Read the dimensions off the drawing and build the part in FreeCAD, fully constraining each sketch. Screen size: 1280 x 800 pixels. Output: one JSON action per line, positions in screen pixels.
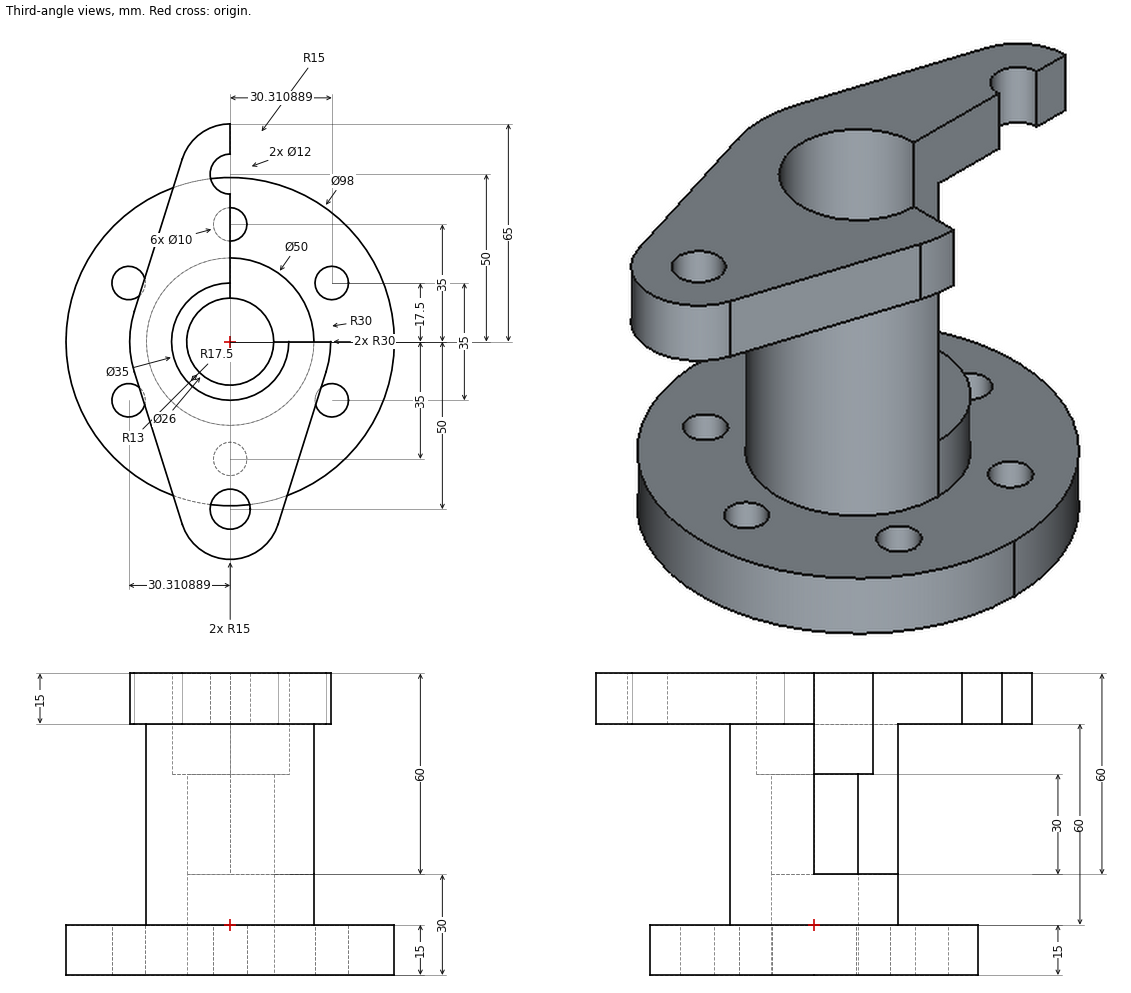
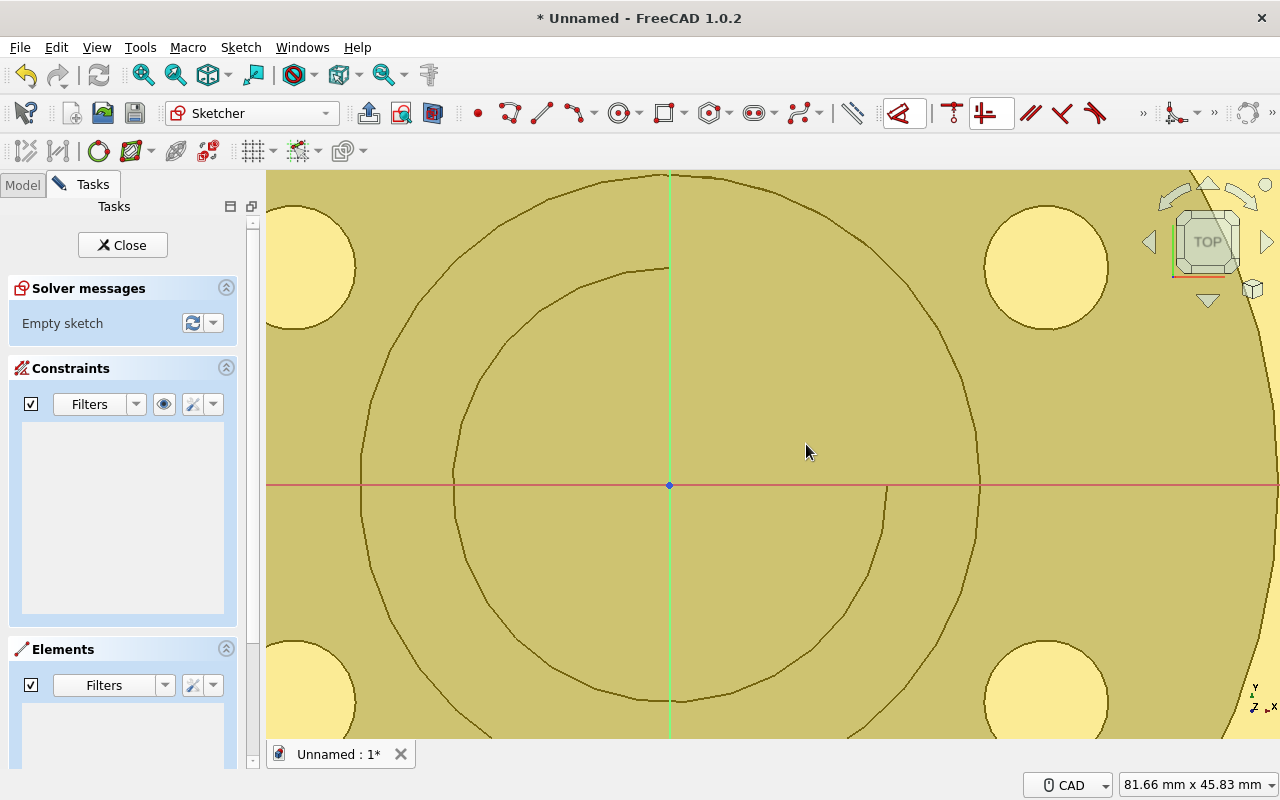
{"action": "left_click", "coordinate": [542, 114]}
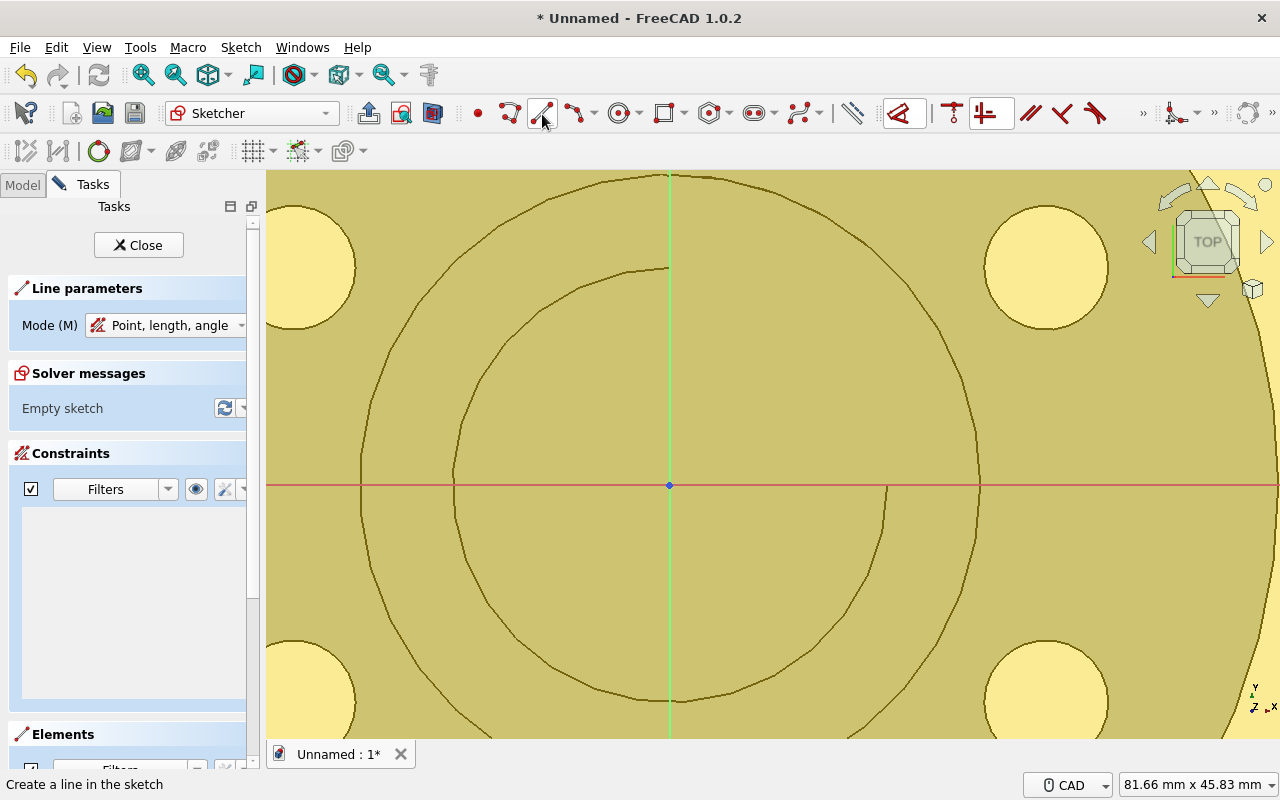
{"action": "left_click", "coordinate": [670, 324]}
{"action": "left_click", "coordinate": [679, 268]}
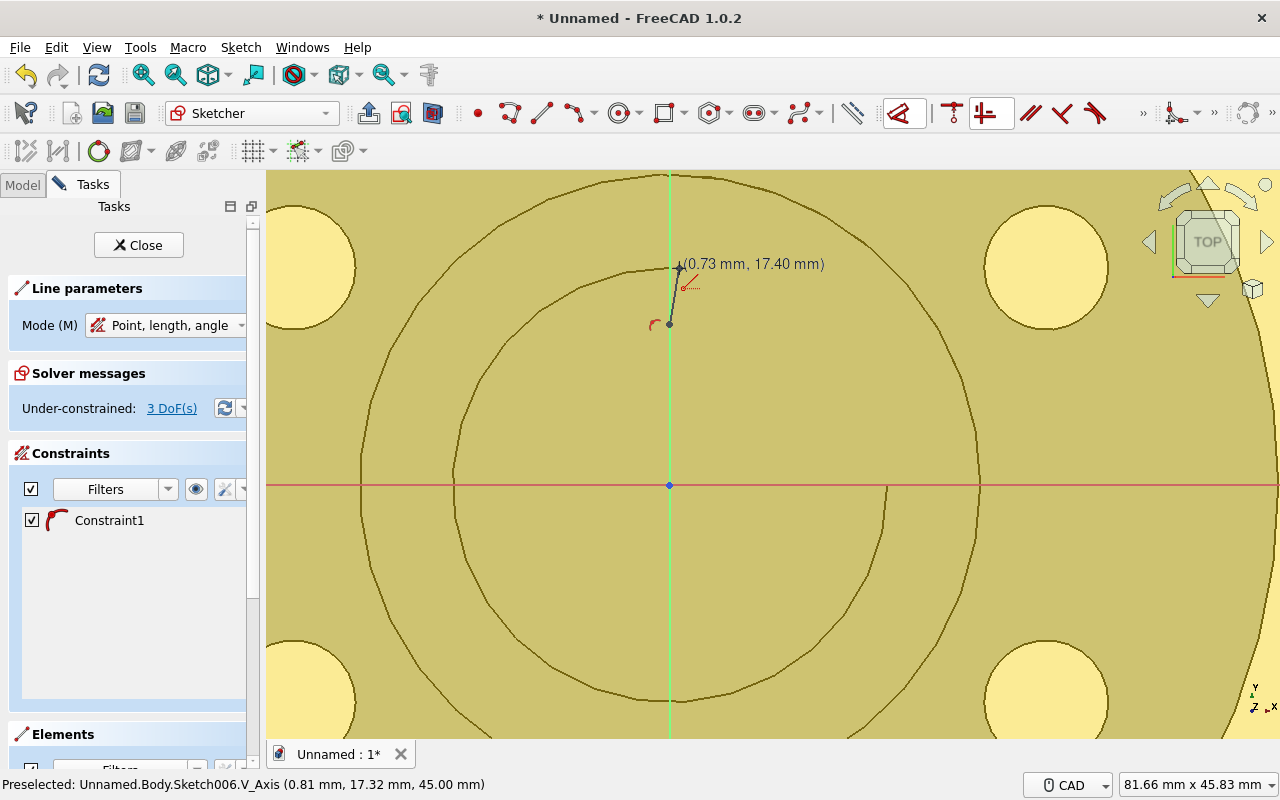
{"action": "left_click", "coordinate": [887, 485]}
{"action": "left_click", "coordinate": [831, 476]}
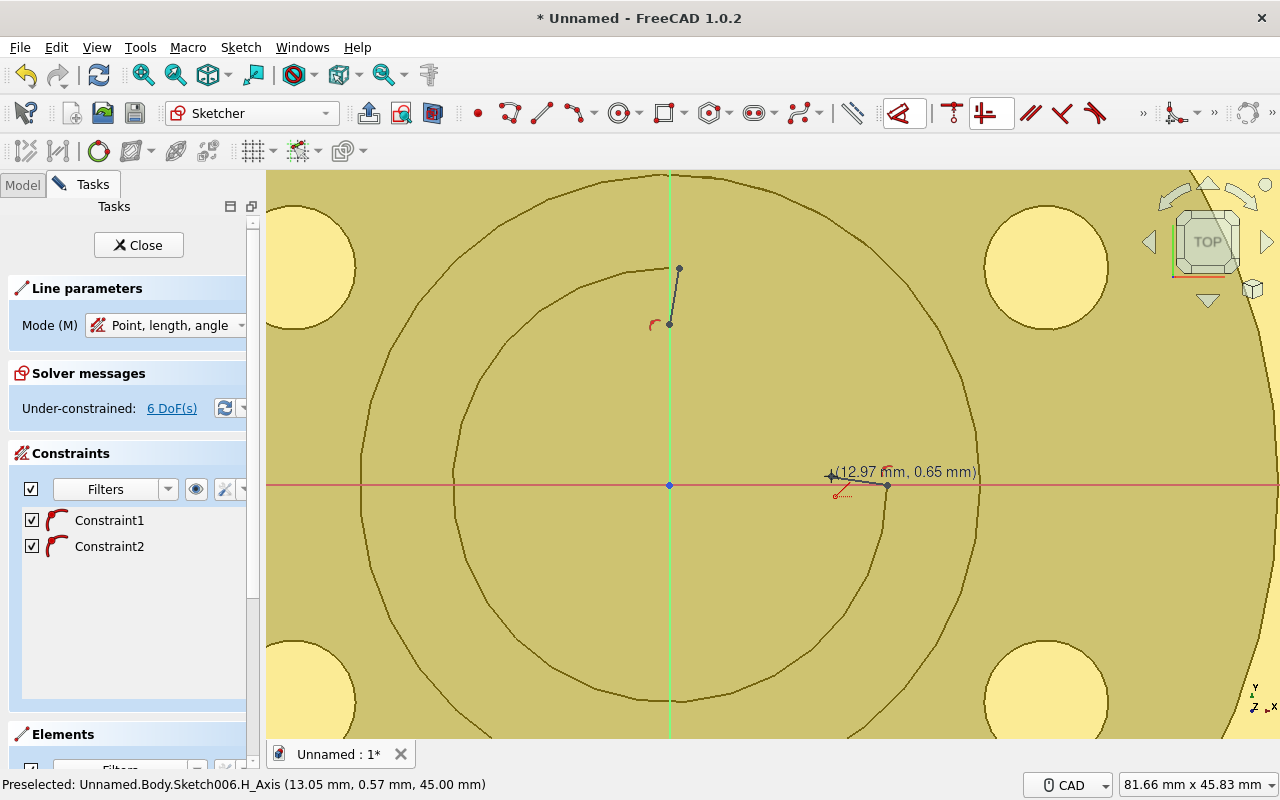
{"action": "left_click", "coordinate": [574, 114]}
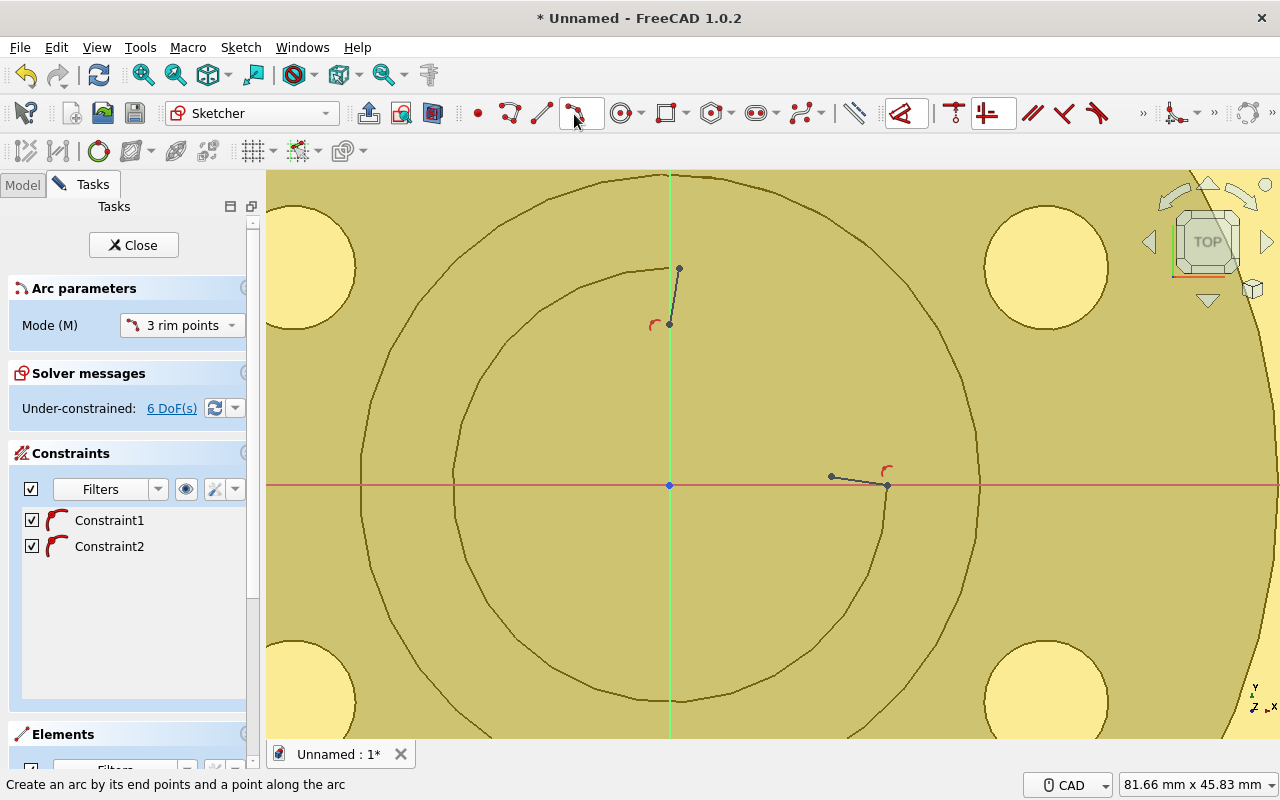
{"action": "left_click", "coordinate": [679, 269]}
{"action": "left_click", "coordinate": [887, 485]}
{"action": "left_click", "coordinate": [516, 639]}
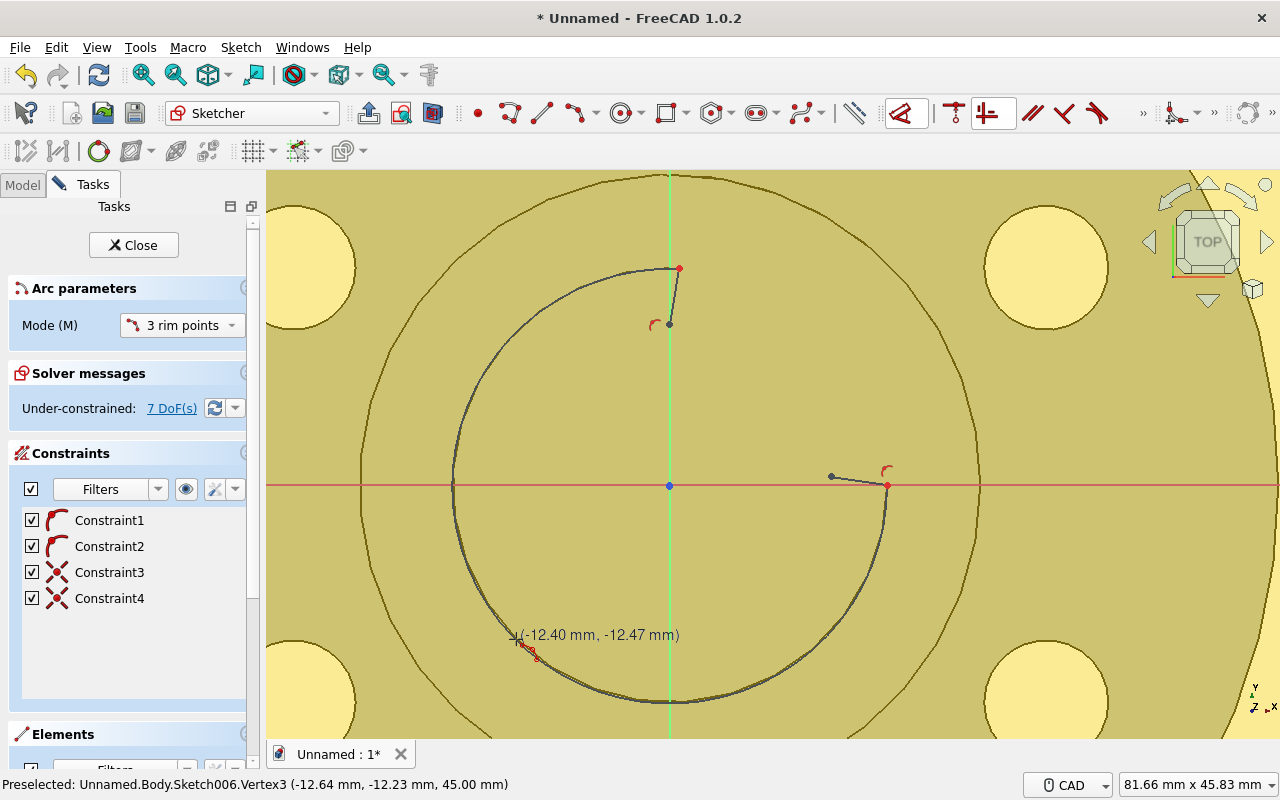
{"action": "left_click", "coordinate": [831, 477]}
{"action": "left_click", "coordinate": [670, 325]}
{"action": "left_click", "coordinate": [556, 599]}
{"action": "key", "text": "Escape"}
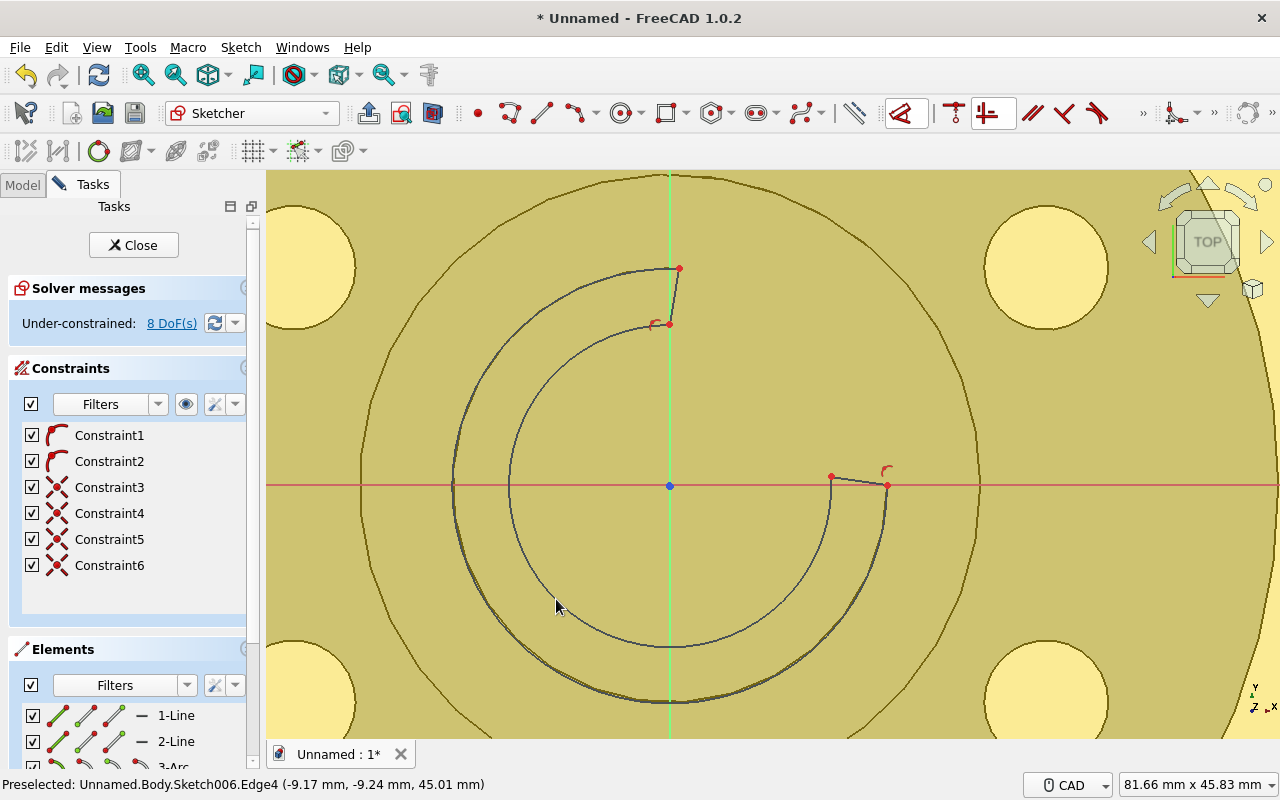
{"action": "left_click", "coordinate": [673, 308]}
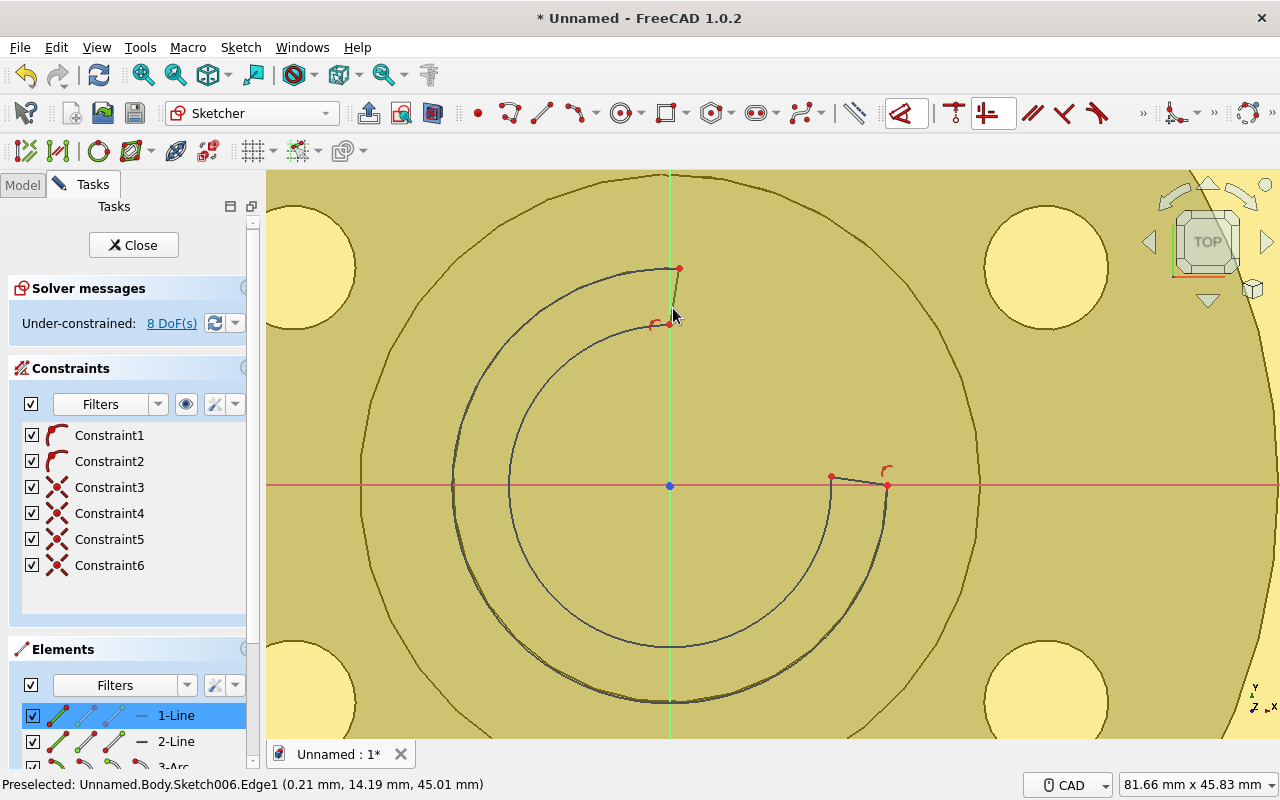
{"action": "key", "text": "v"}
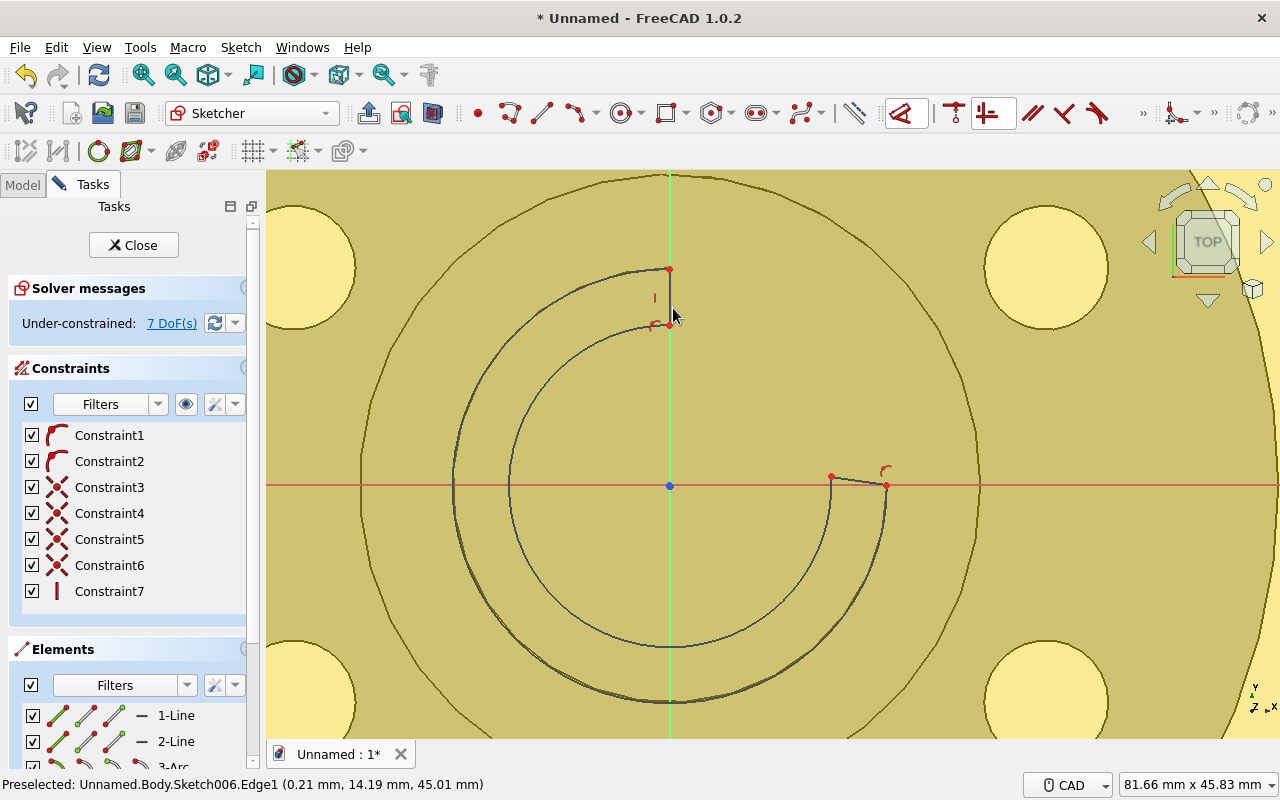
{"action": "left_click", "coordinate": [870, 483]}